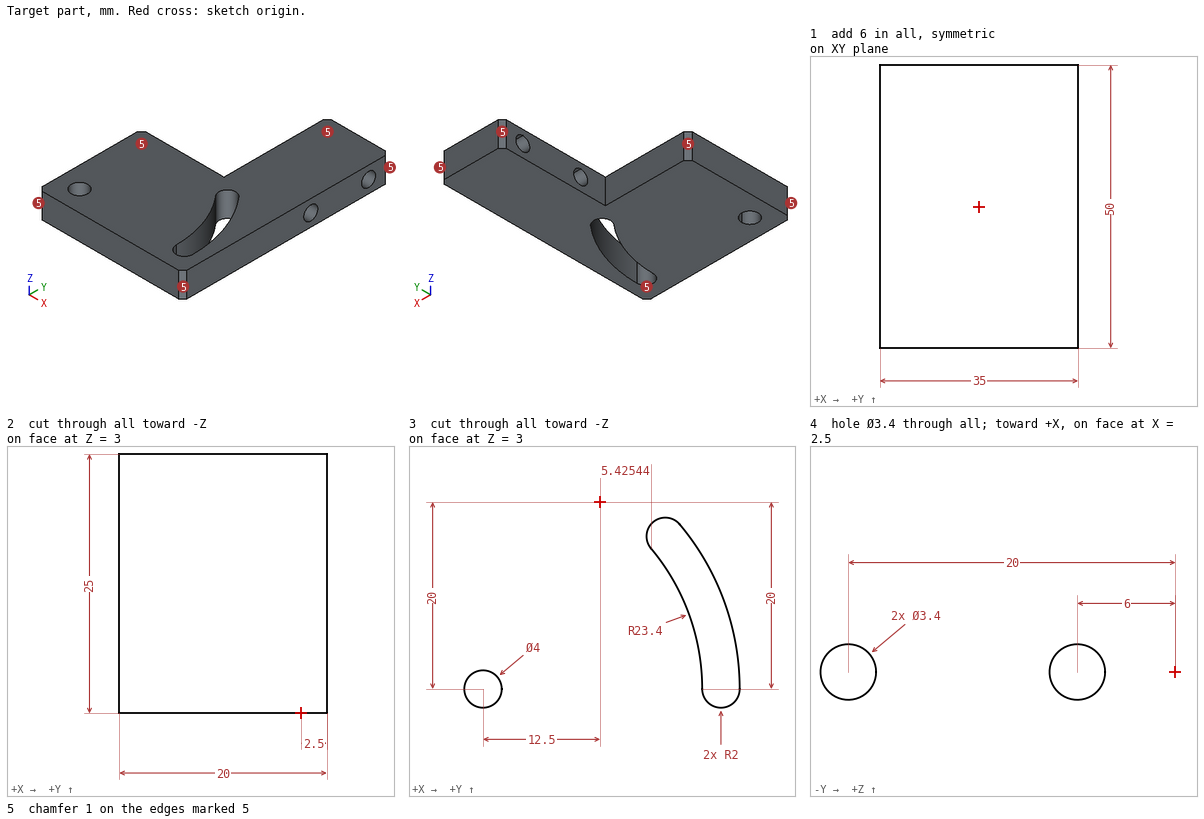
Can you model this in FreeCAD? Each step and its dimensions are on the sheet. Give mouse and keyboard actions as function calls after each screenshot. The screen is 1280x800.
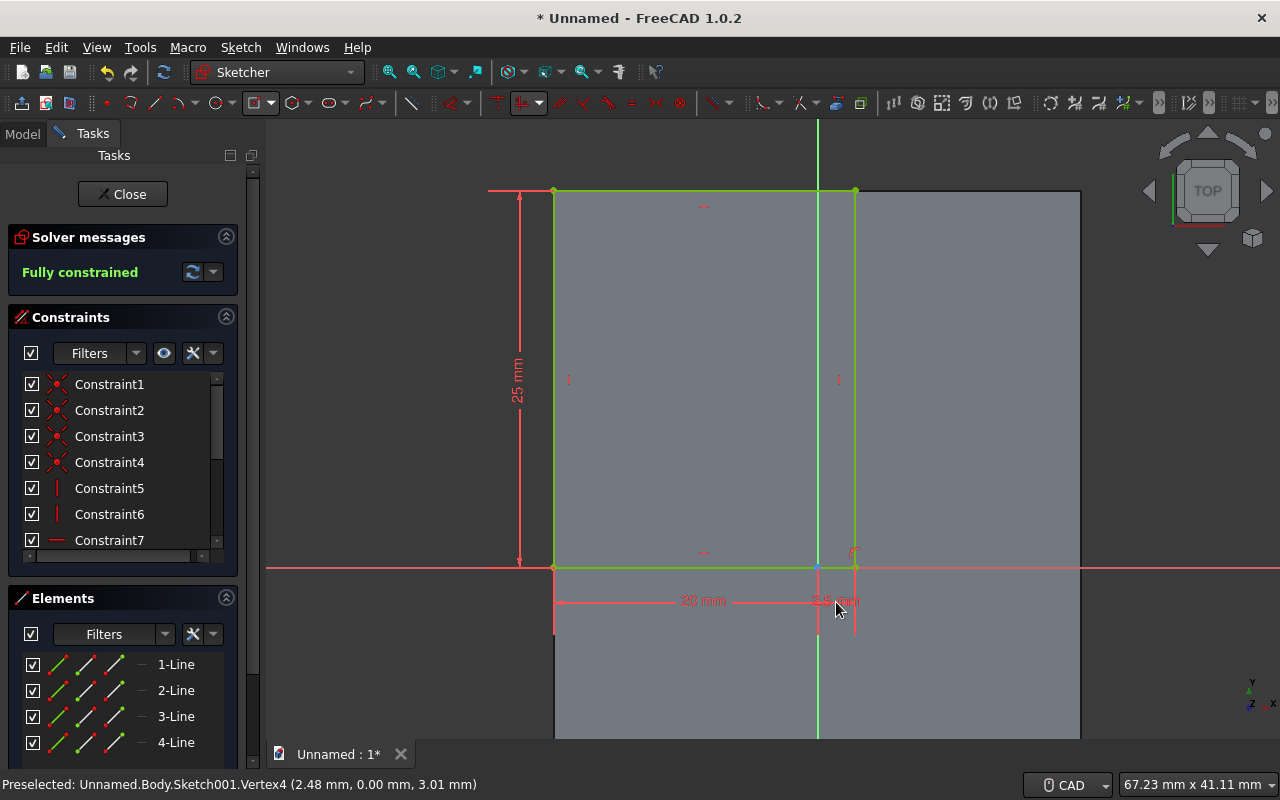
click(123, 194)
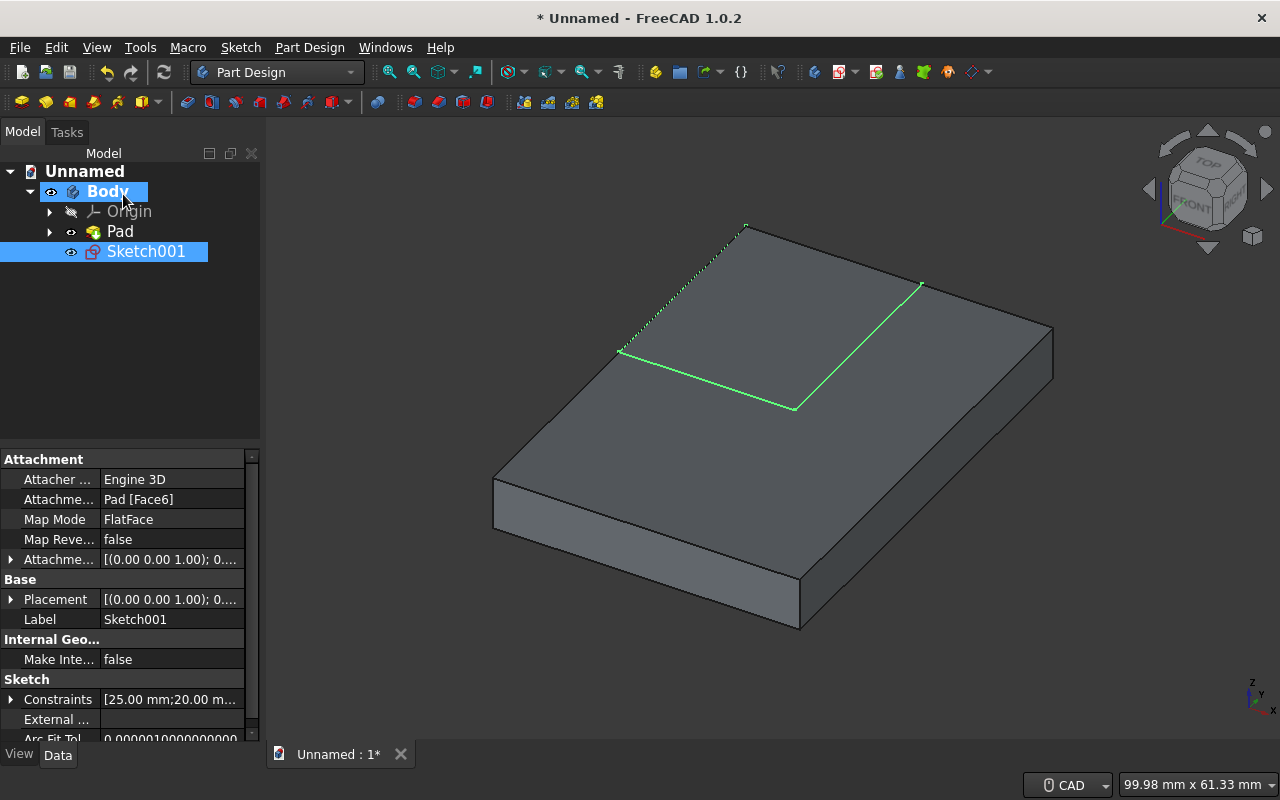
click(188, 102)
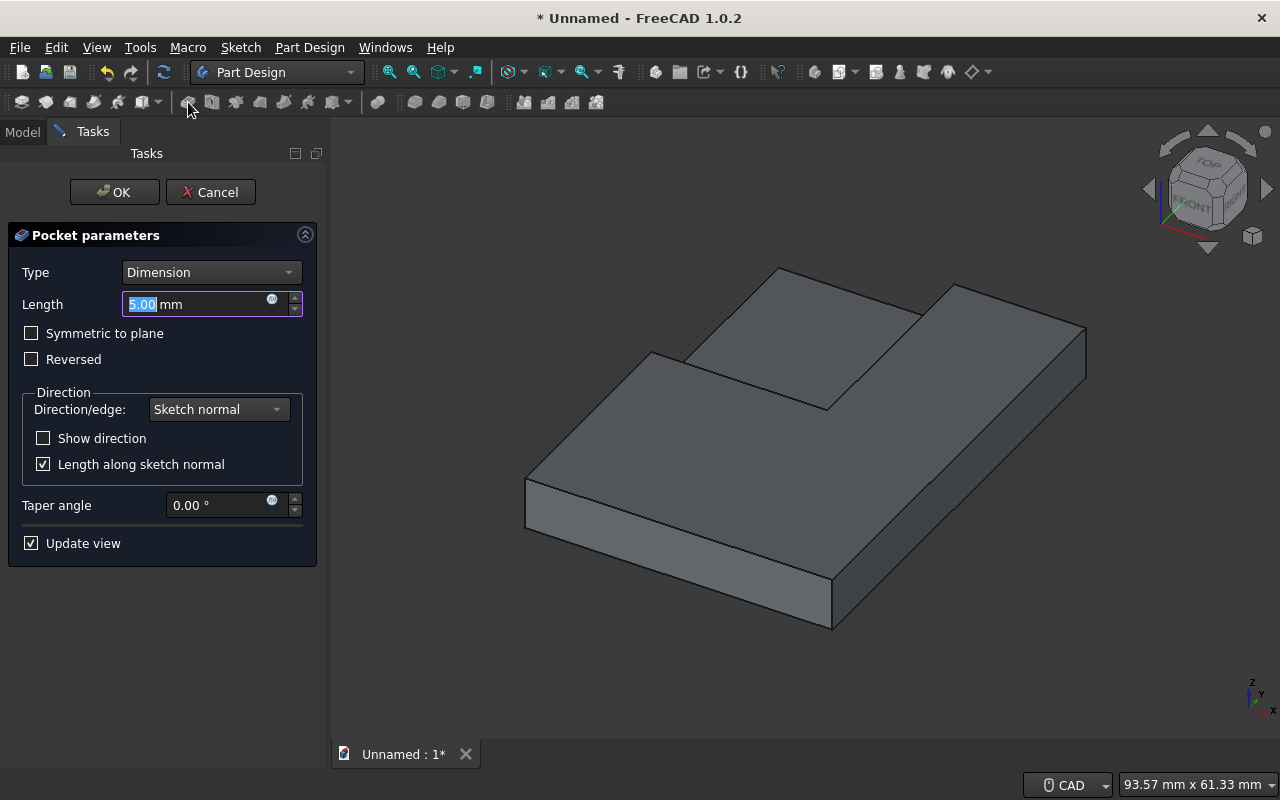
click(212, 272)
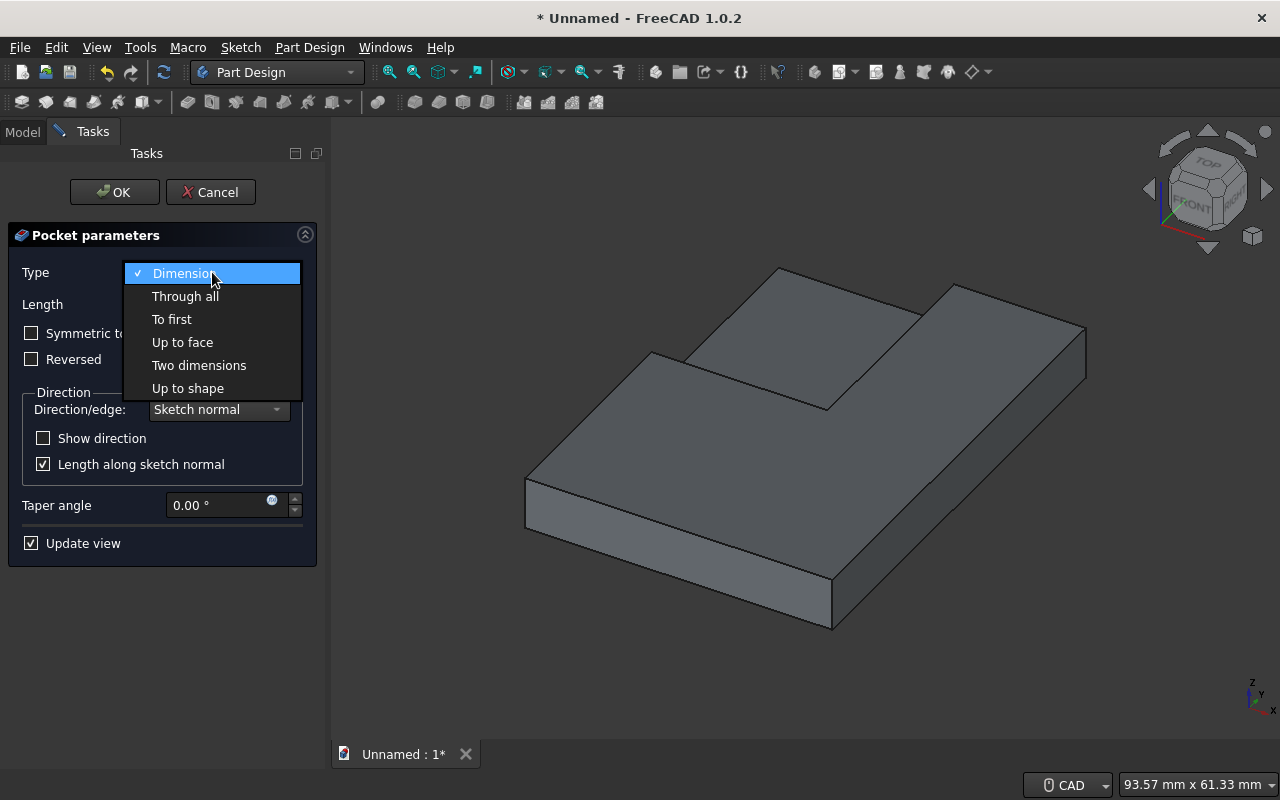
click(212, 296)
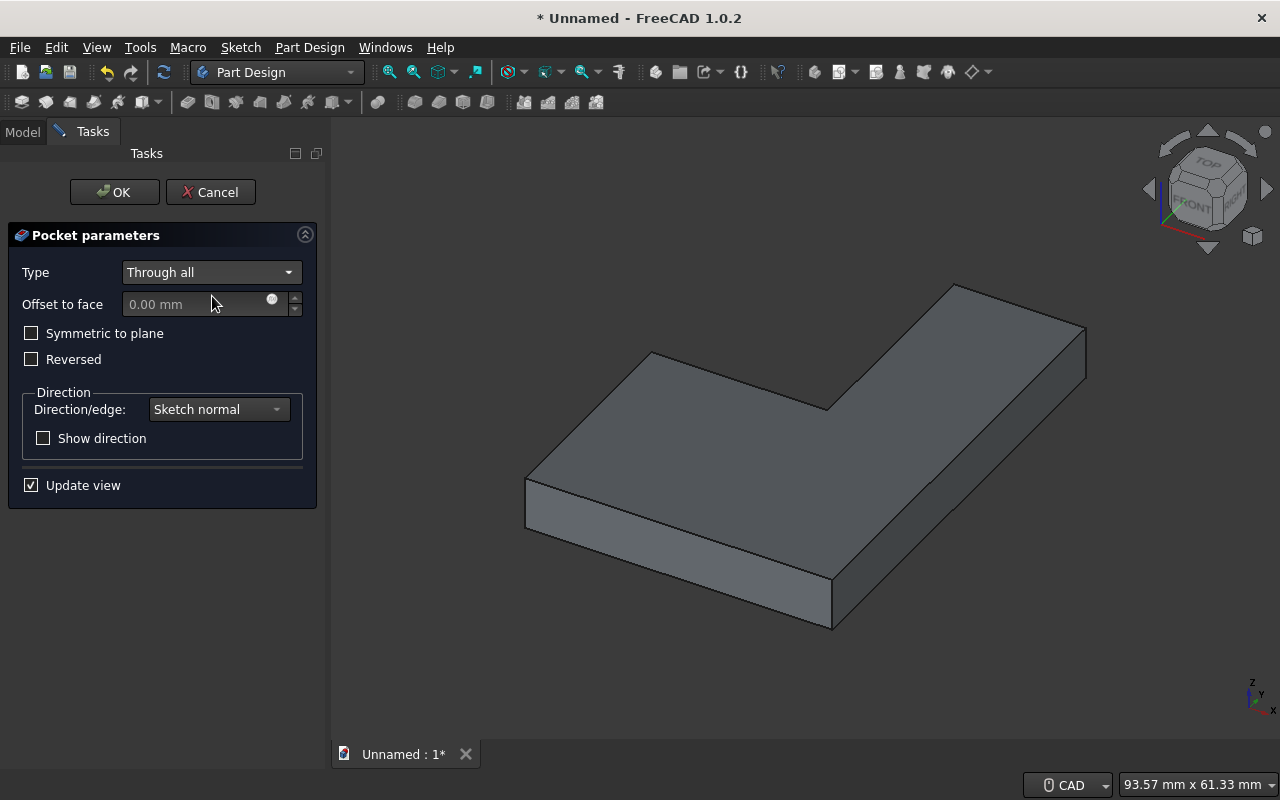
click(115, 192)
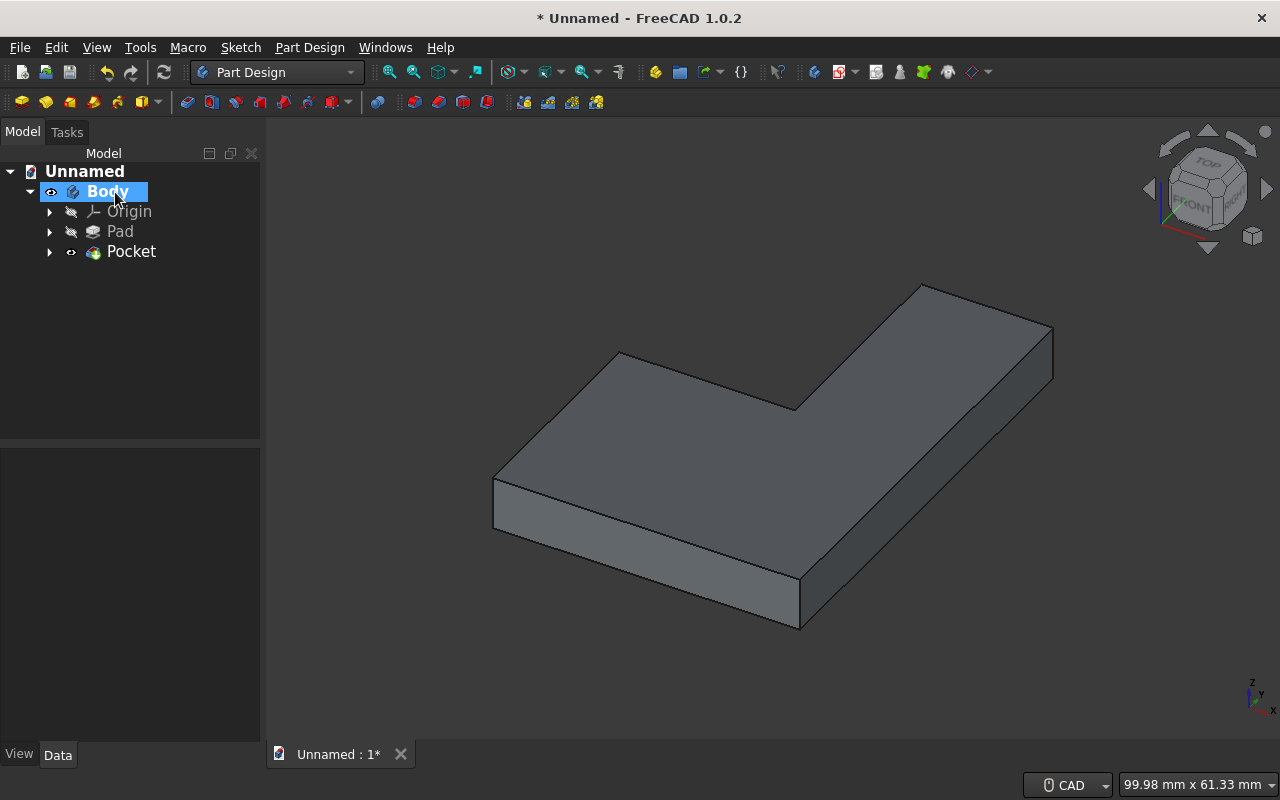
click(744, 489)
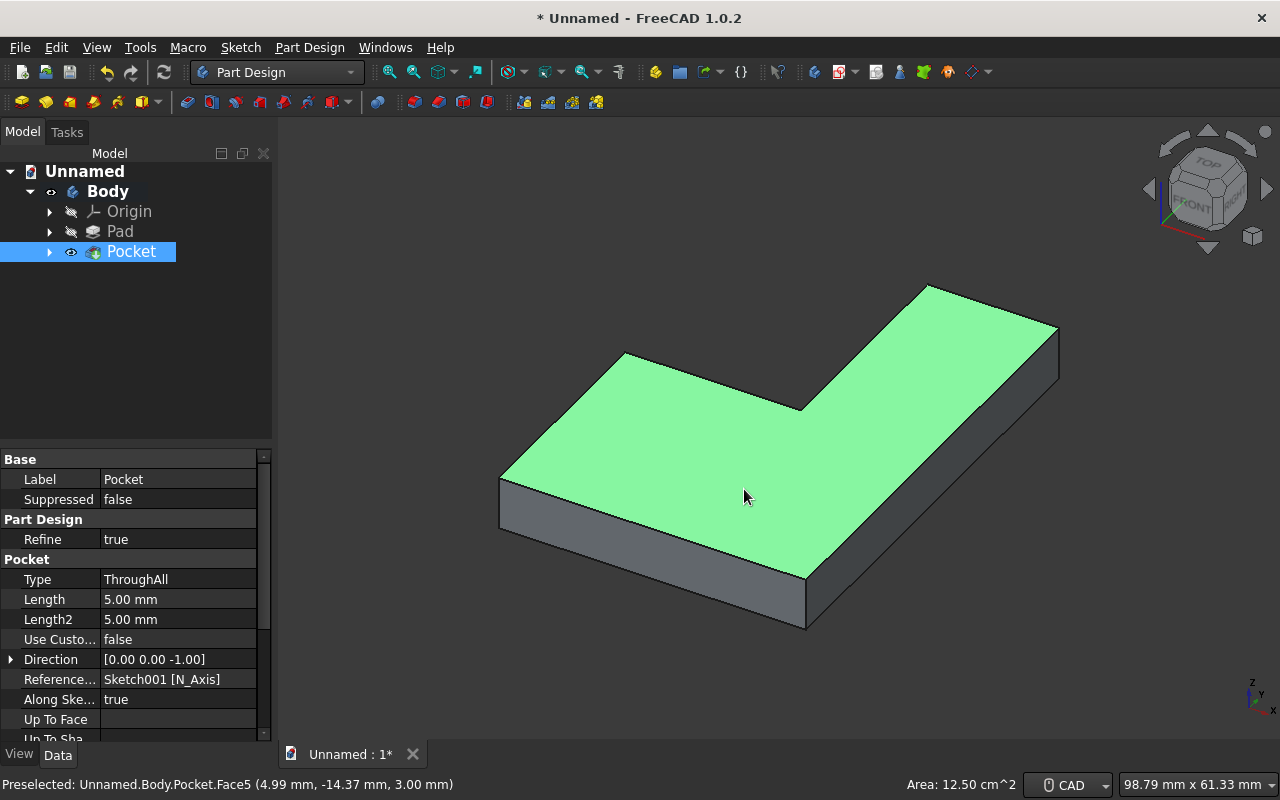
click(840, 72)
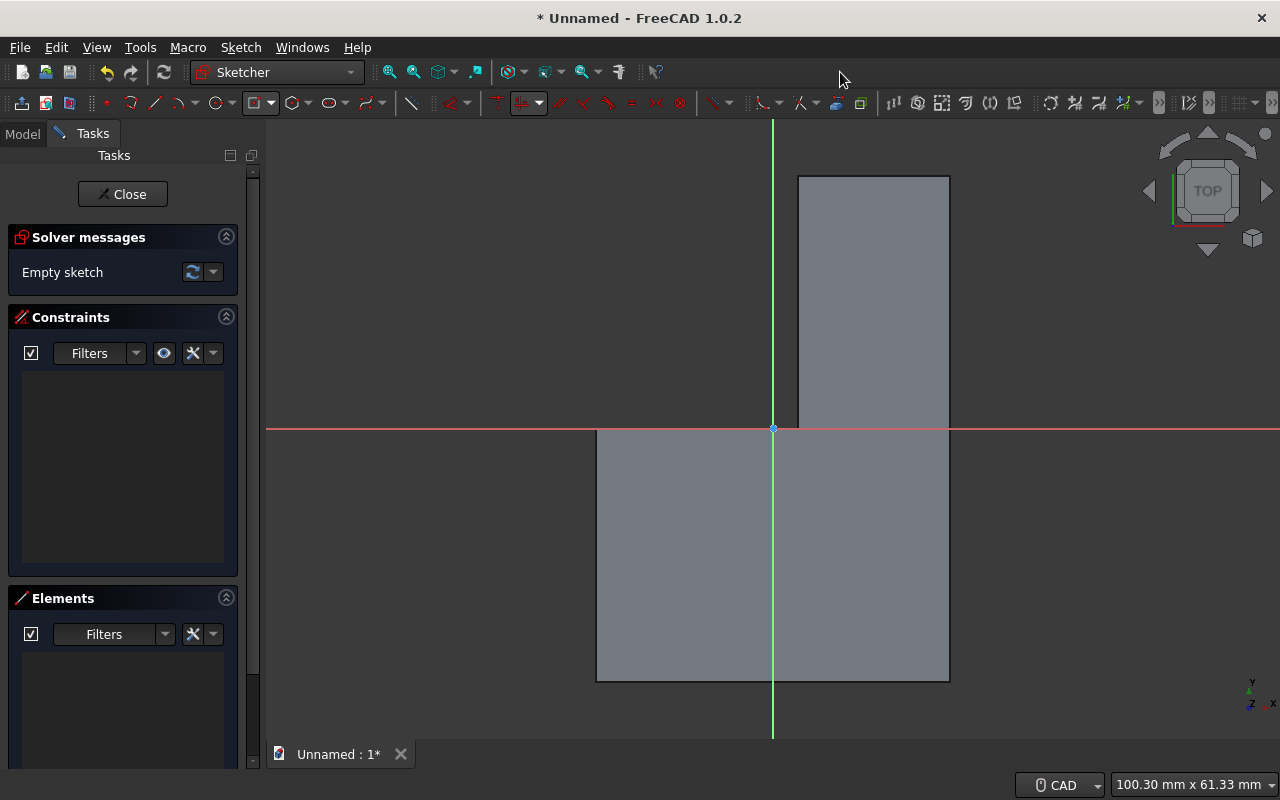
scroll(861, 675, up, 3)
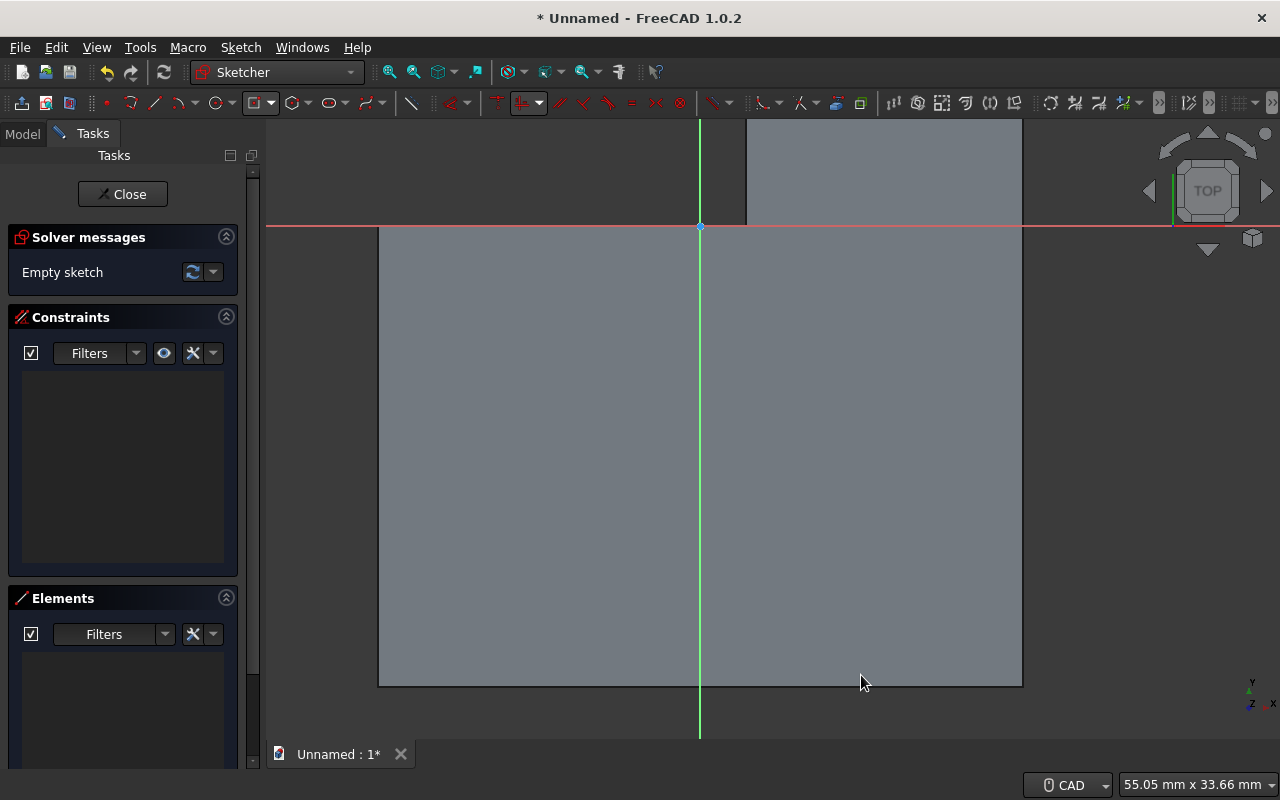
click(198, 104)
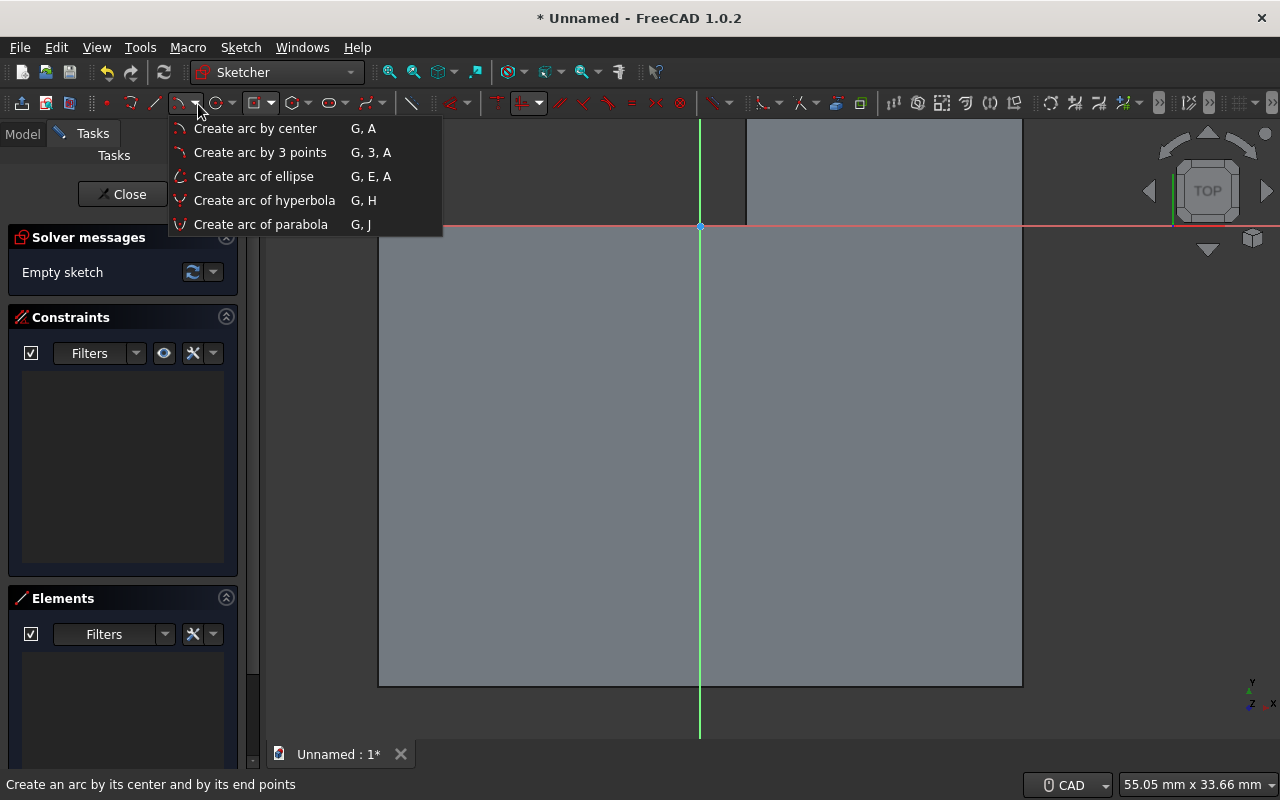
click(306, 152)